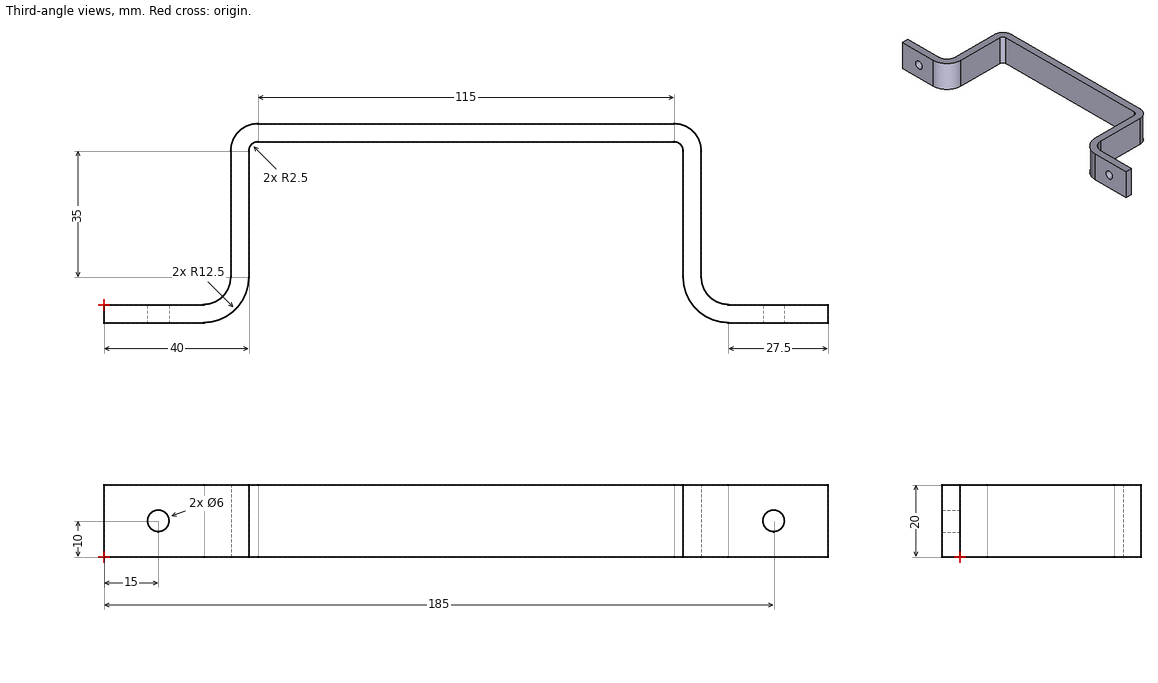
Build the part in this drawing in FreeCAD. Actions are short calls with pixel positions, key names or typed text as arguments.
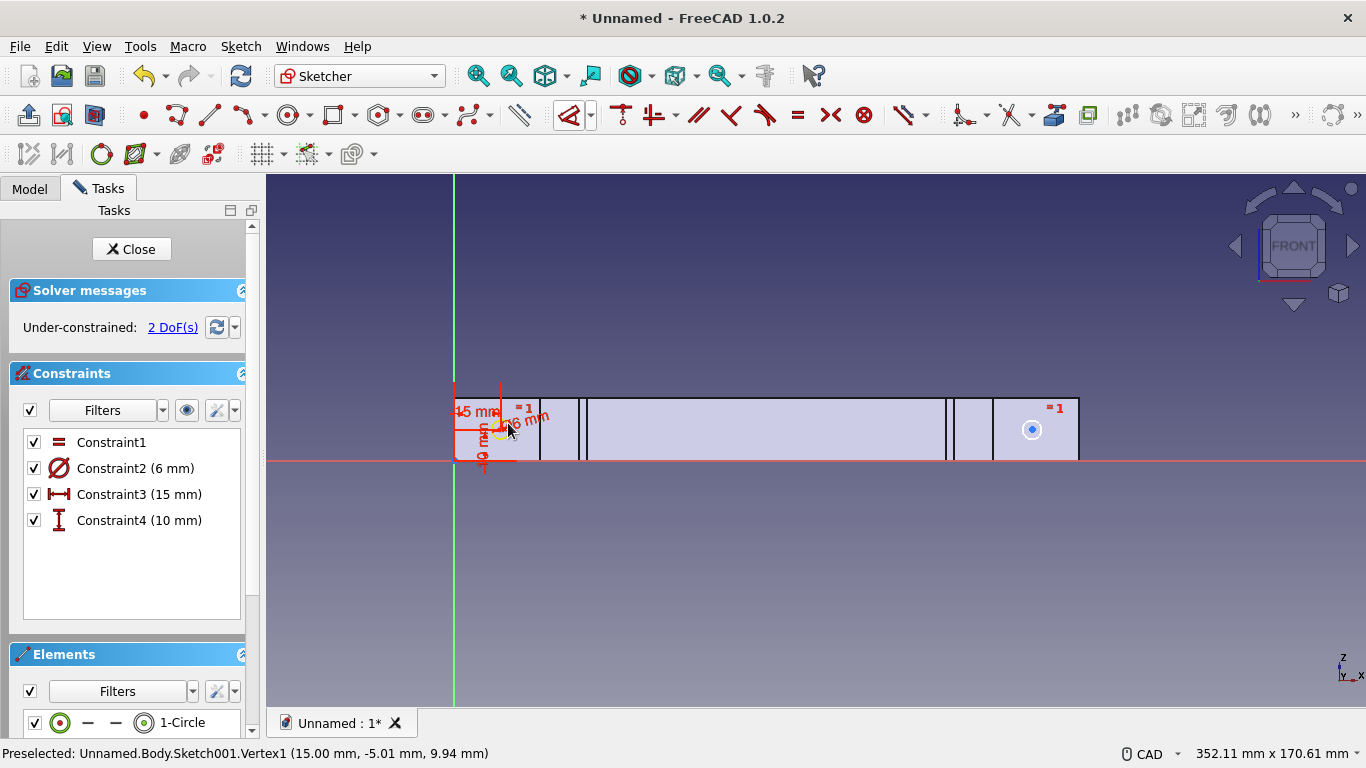
scroll(1032, 430, up, 2)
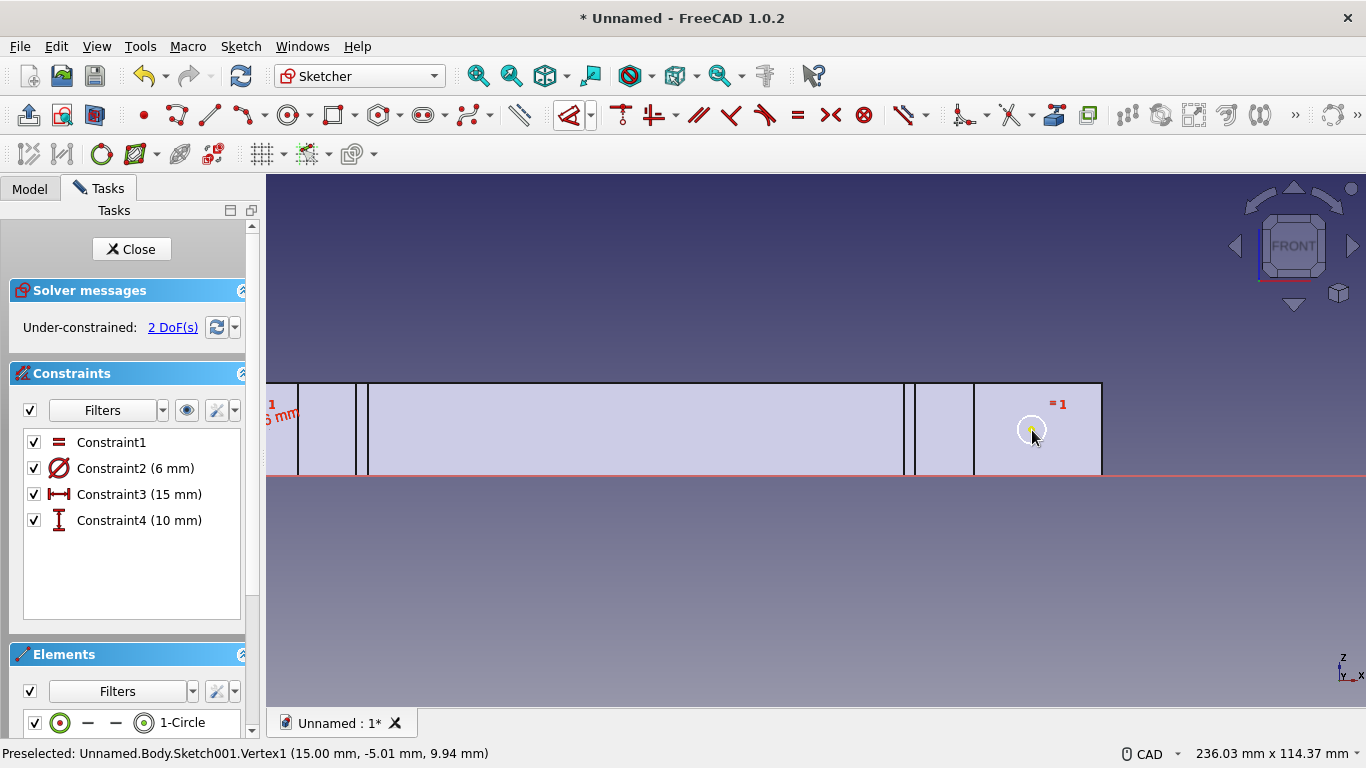
click(1032, 430)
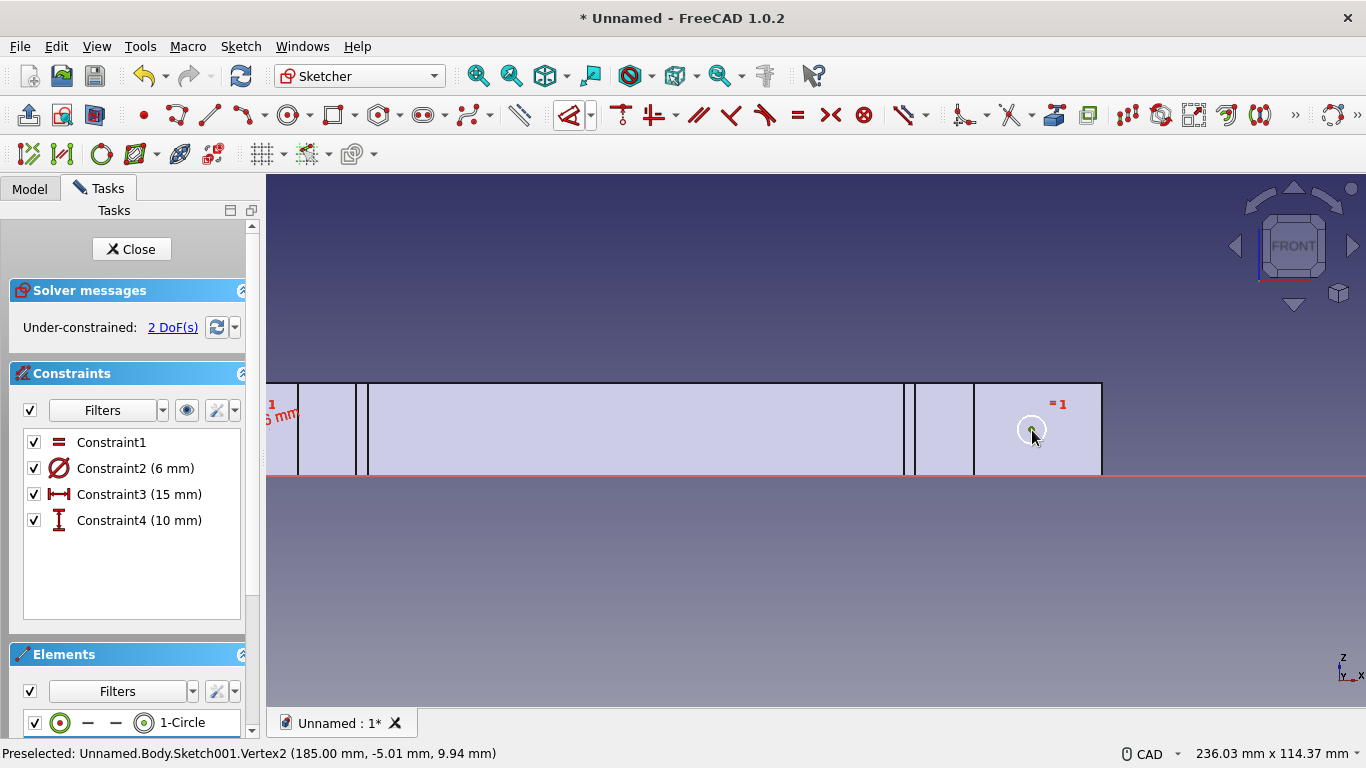
click(590, 116)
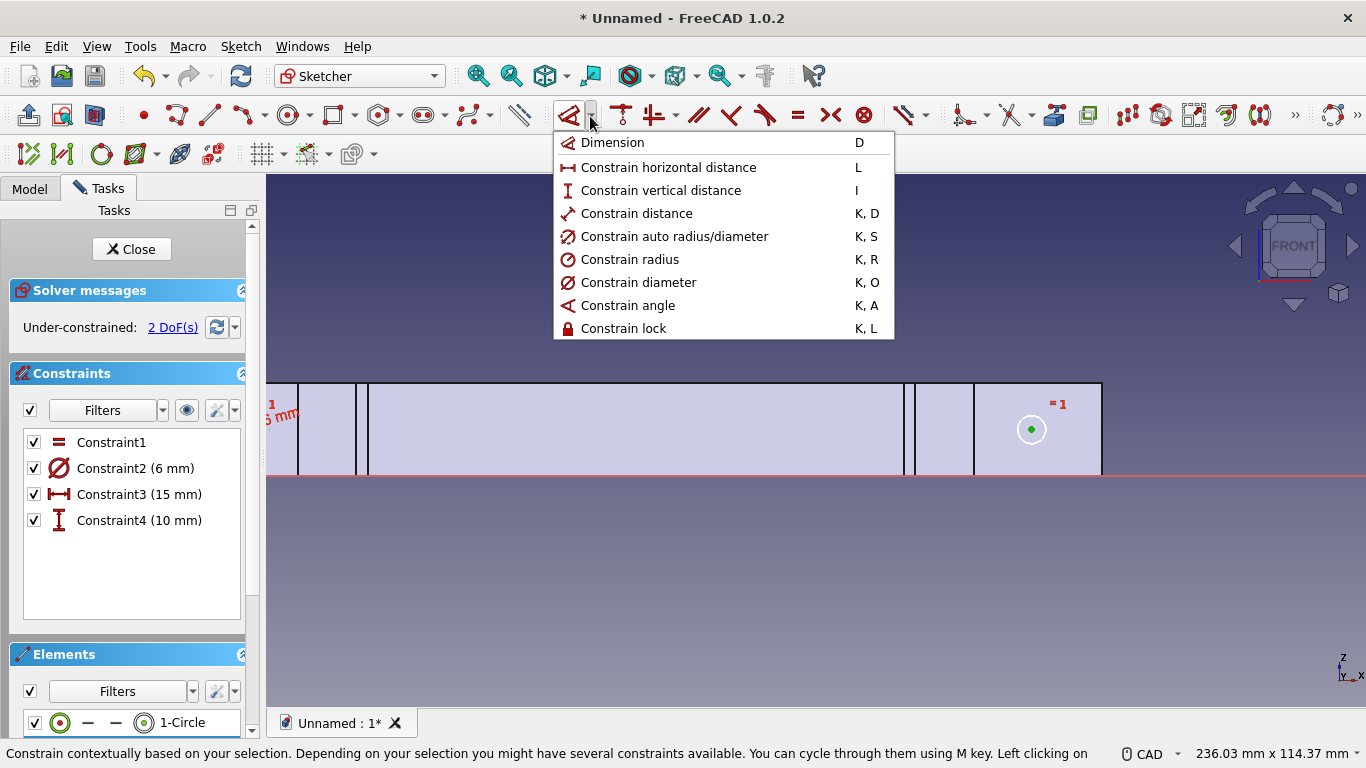
click(724, 190)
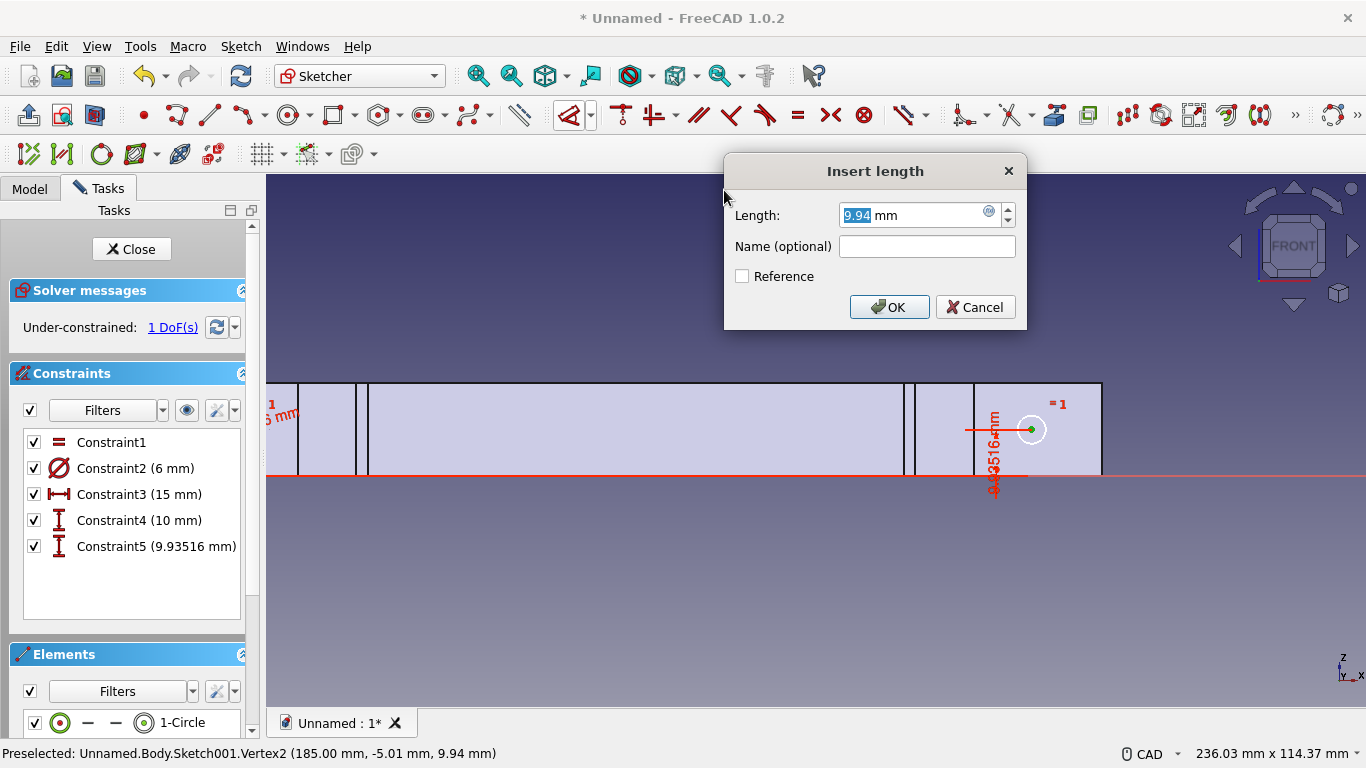
text(10)
key(Return)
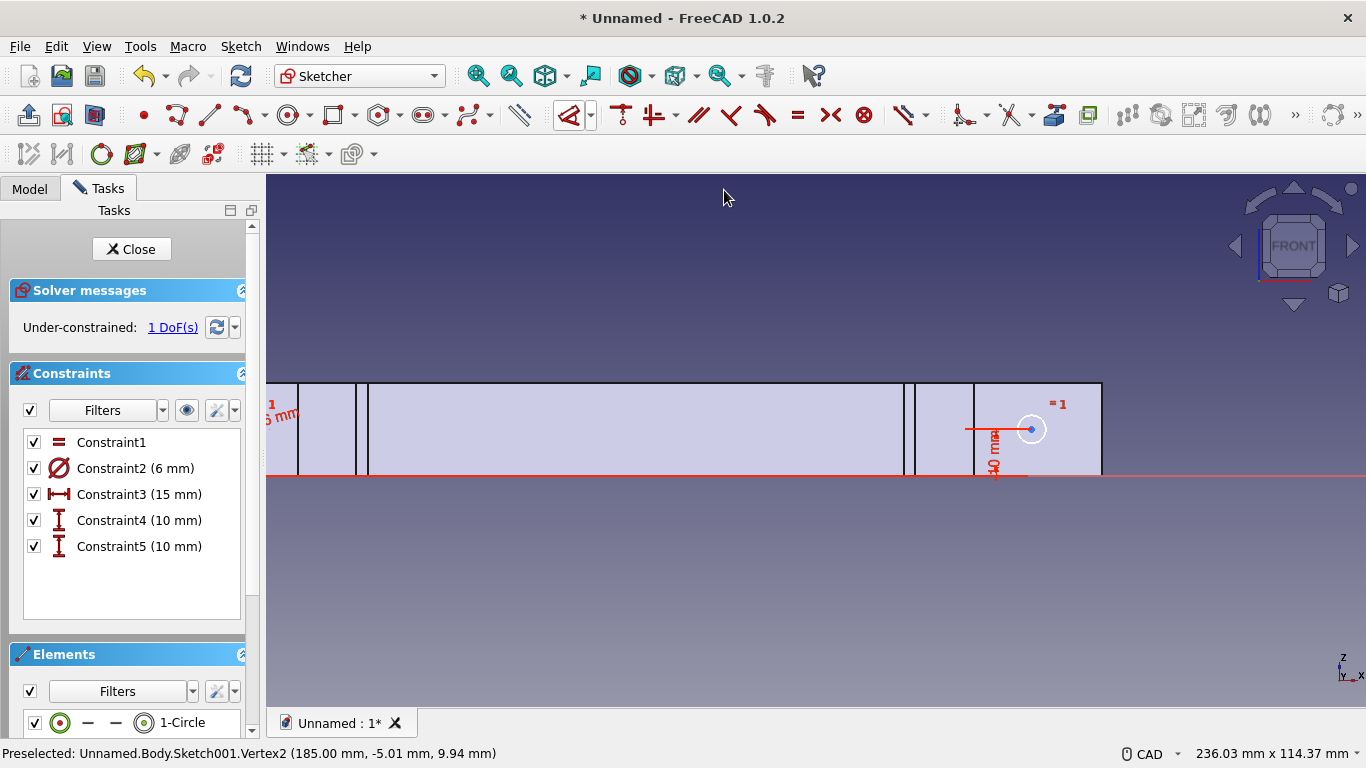
click(1032, 429)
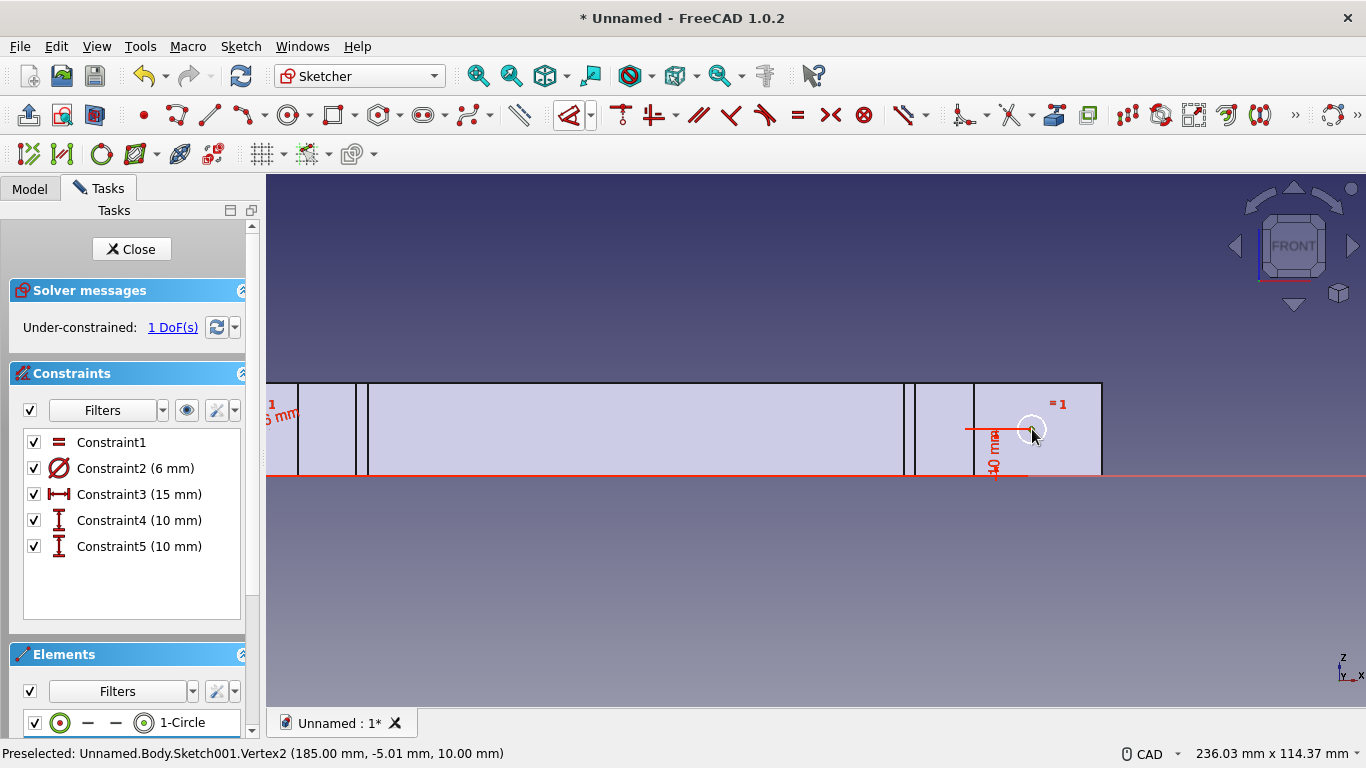
key(l)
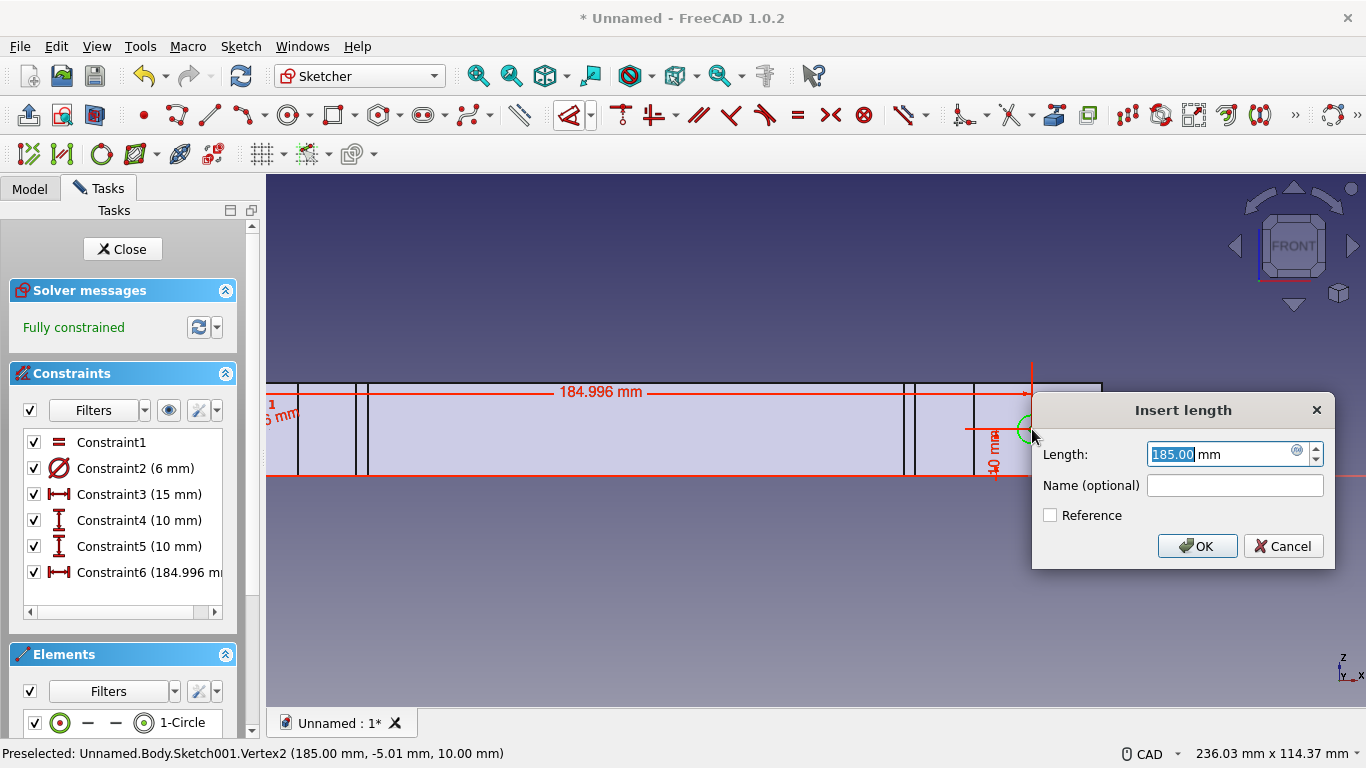
text(185)
key(Return)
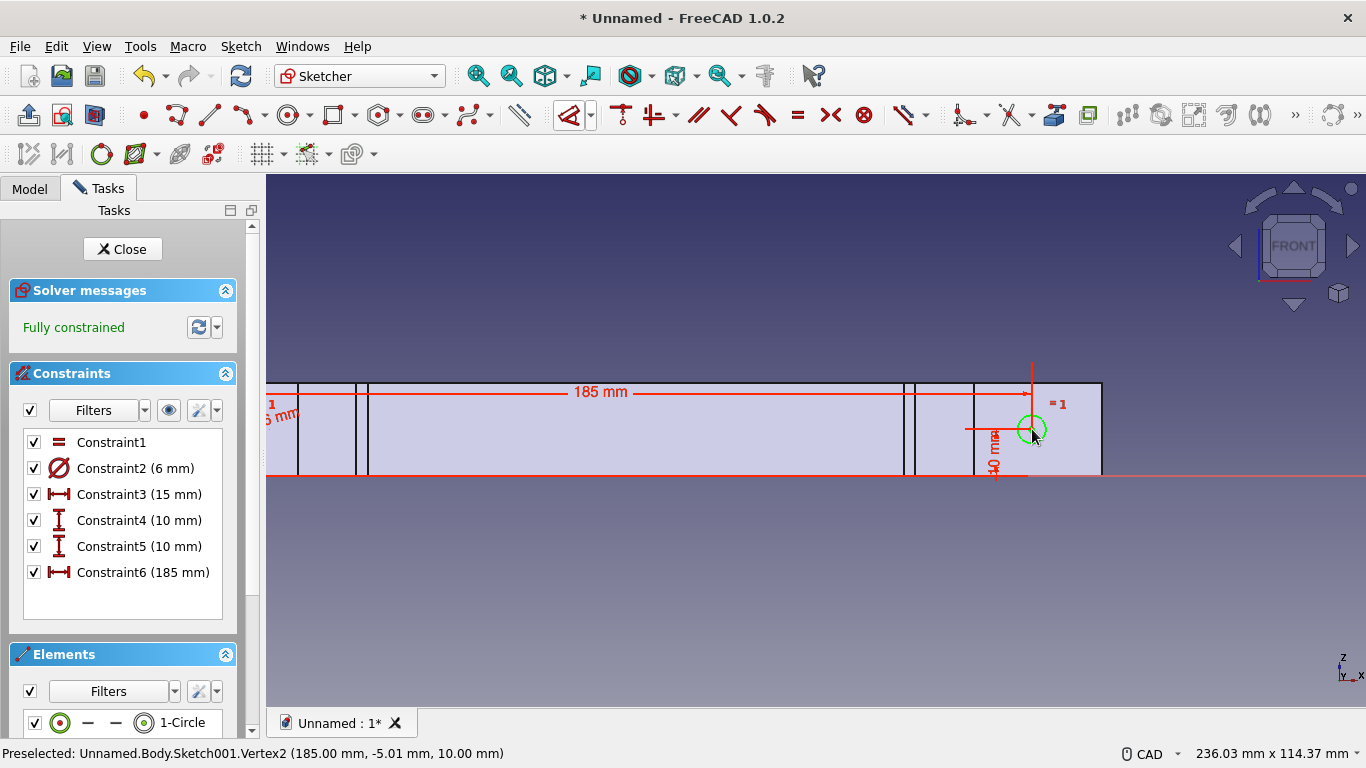
click(123, 249)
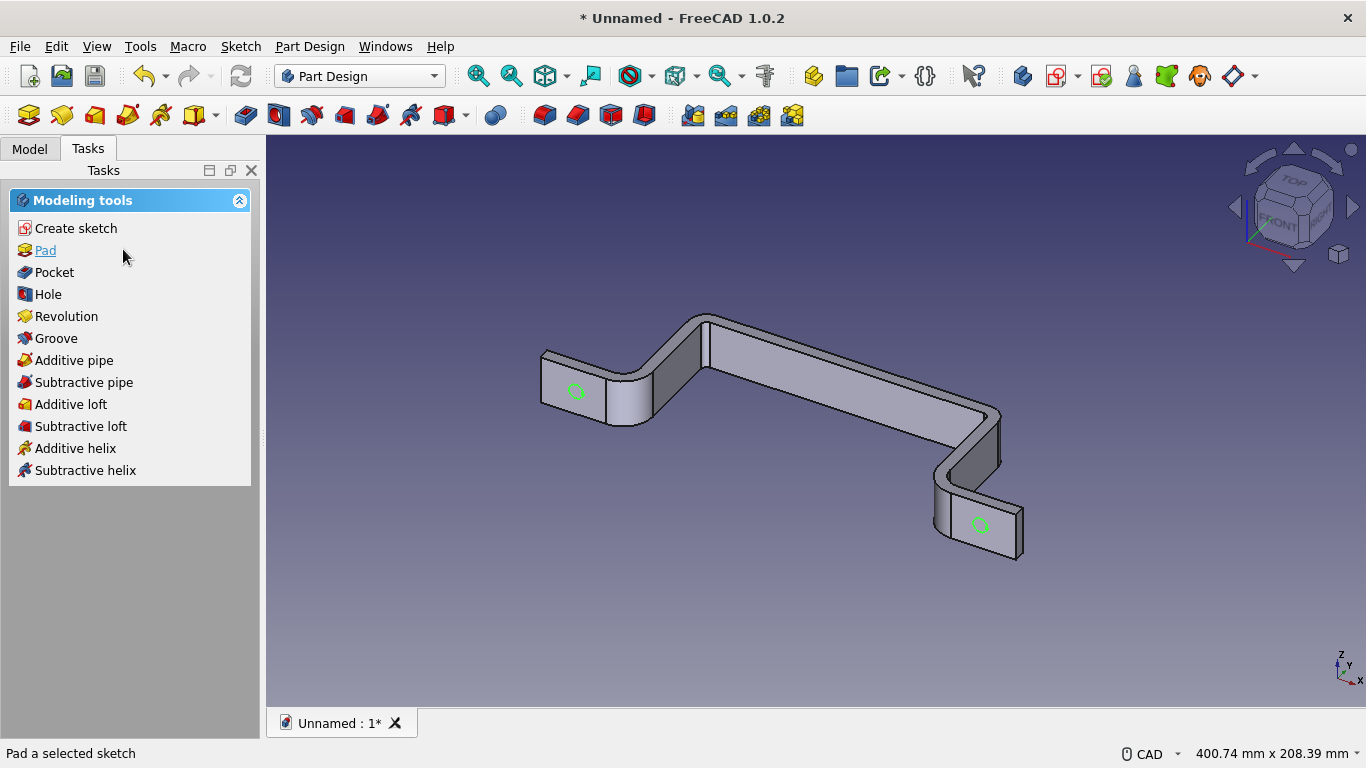
click(246, 116)